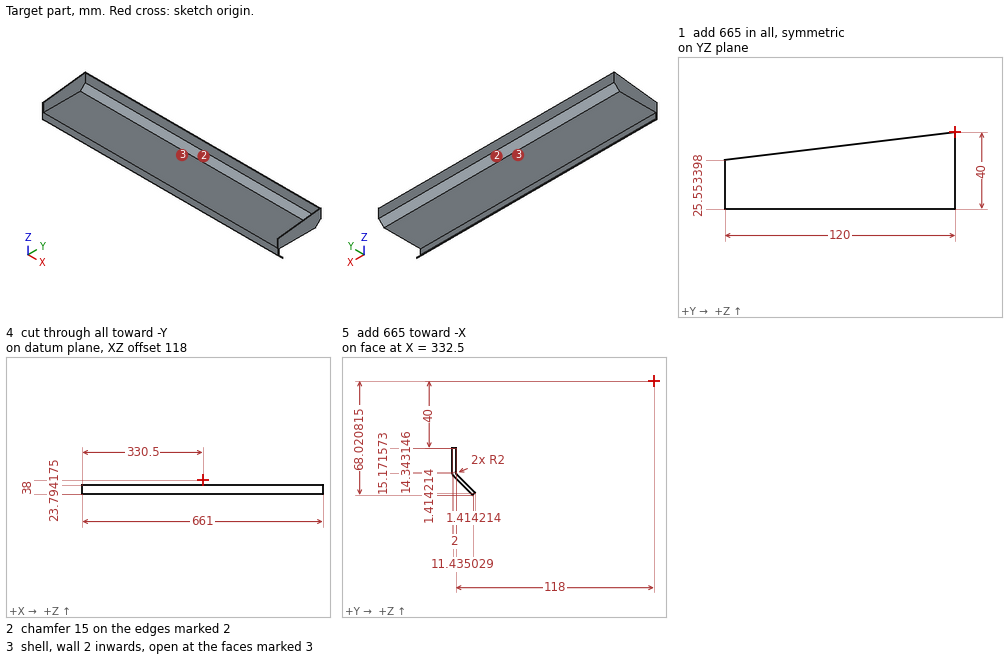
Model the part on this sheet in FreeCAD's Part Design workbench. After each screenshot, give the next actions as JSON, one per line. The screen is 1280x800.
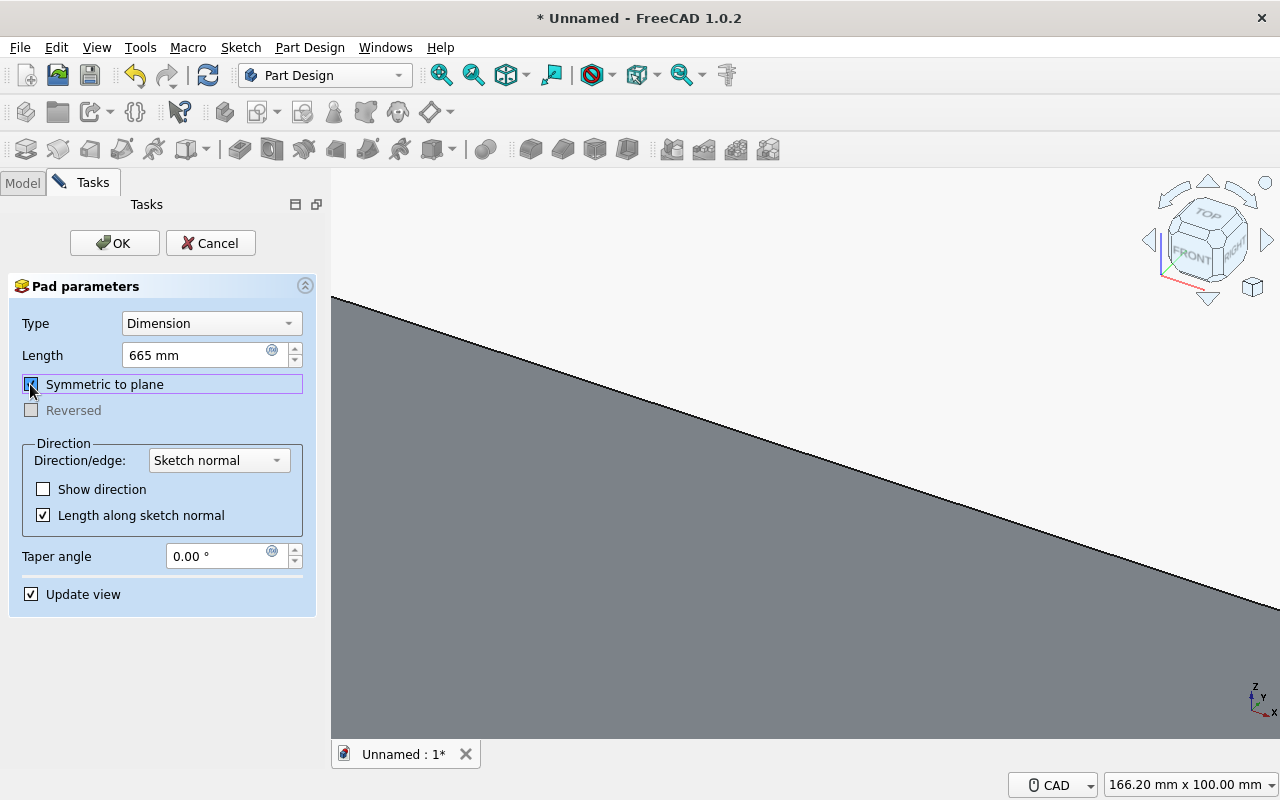
{"action": "left_click", "coordinate": [115, 243]}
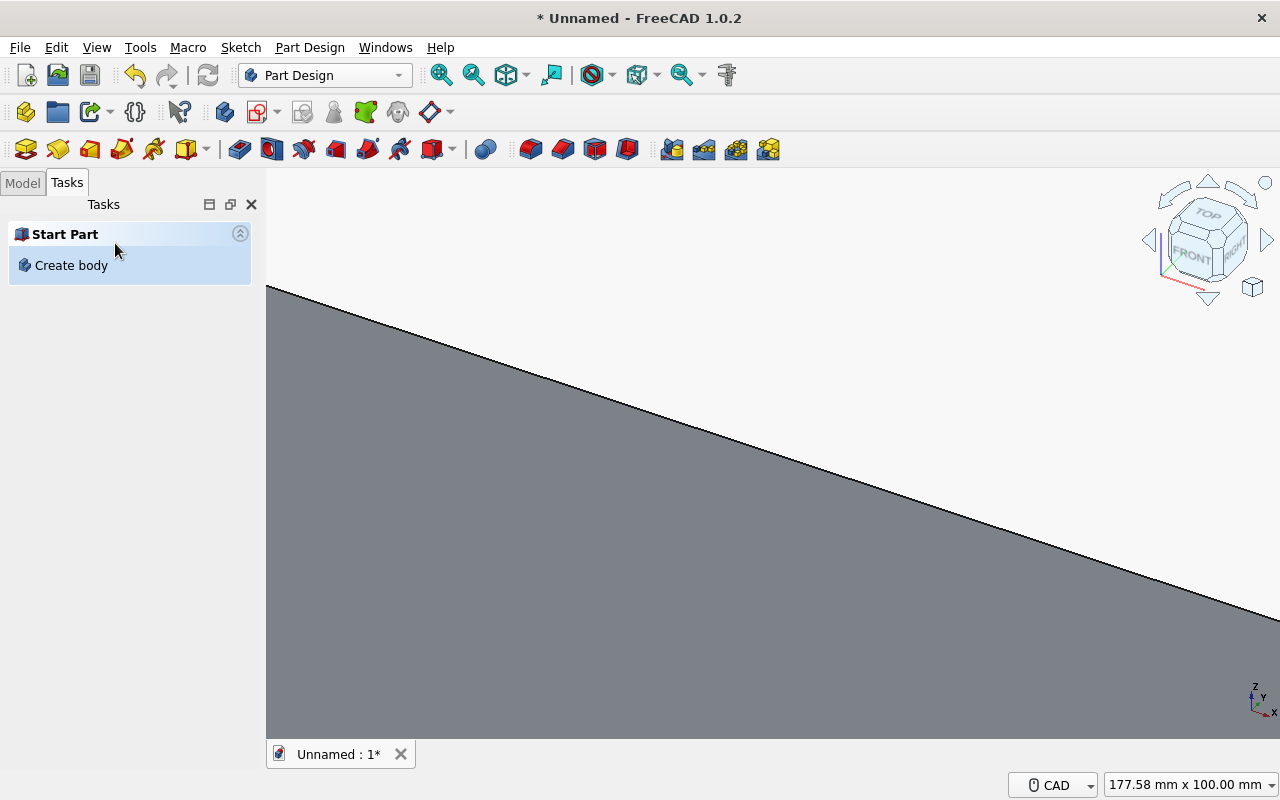
{"action": "left_click", "coordinate": [442, 76]}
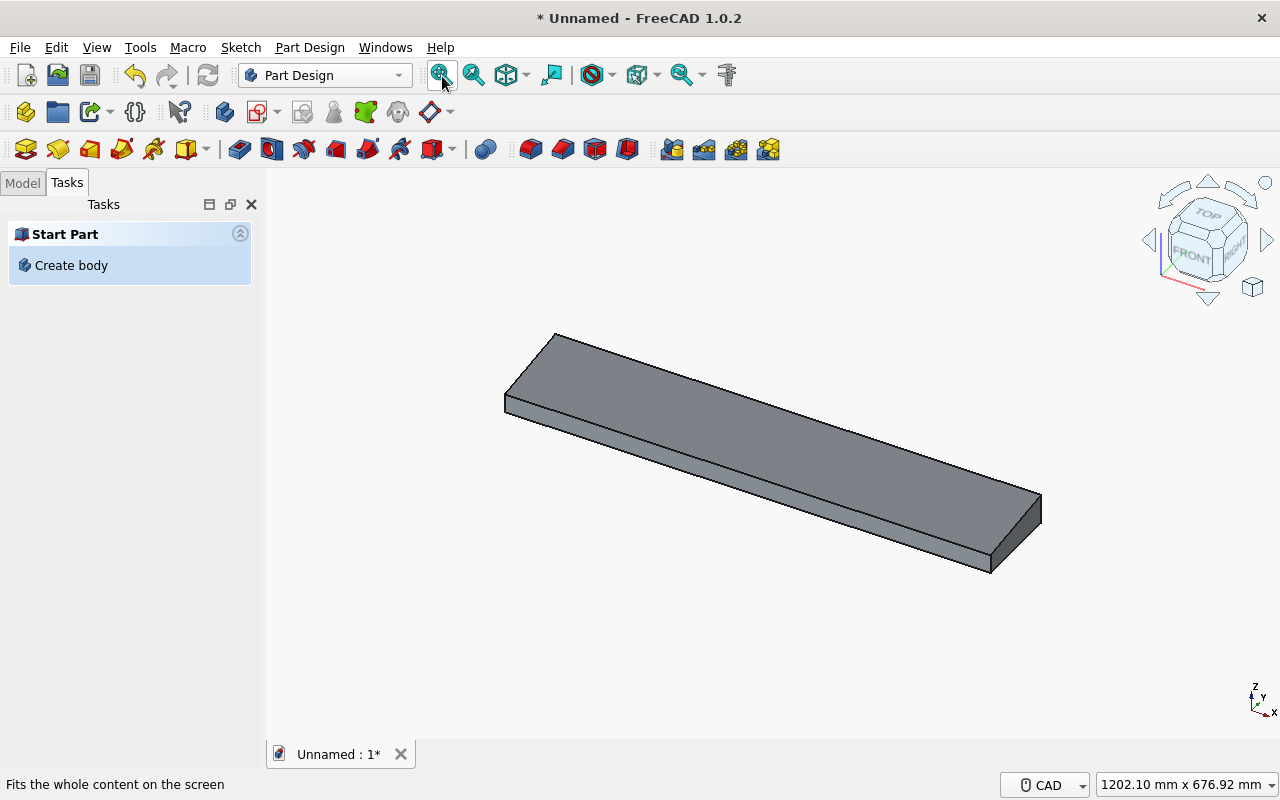
{"action": "key", "text": "0"}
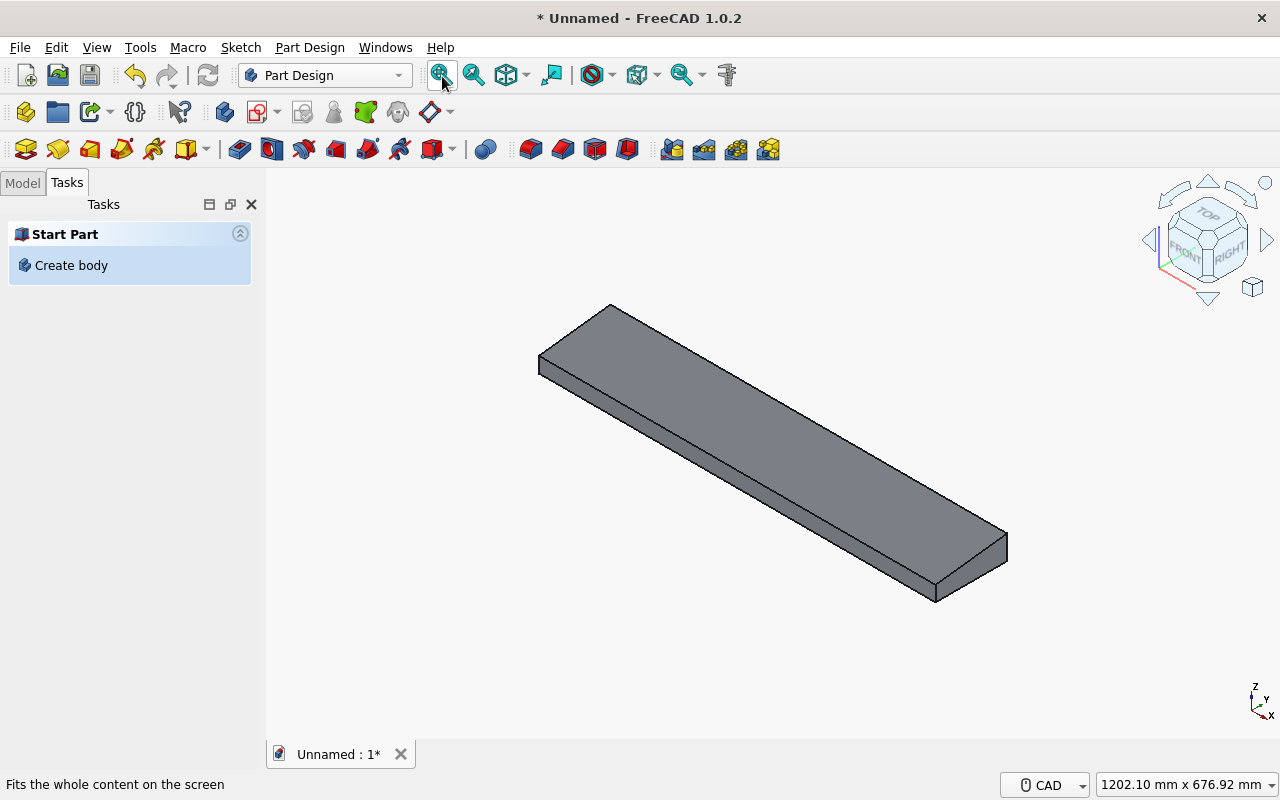
{"action": "key", "text": "2"}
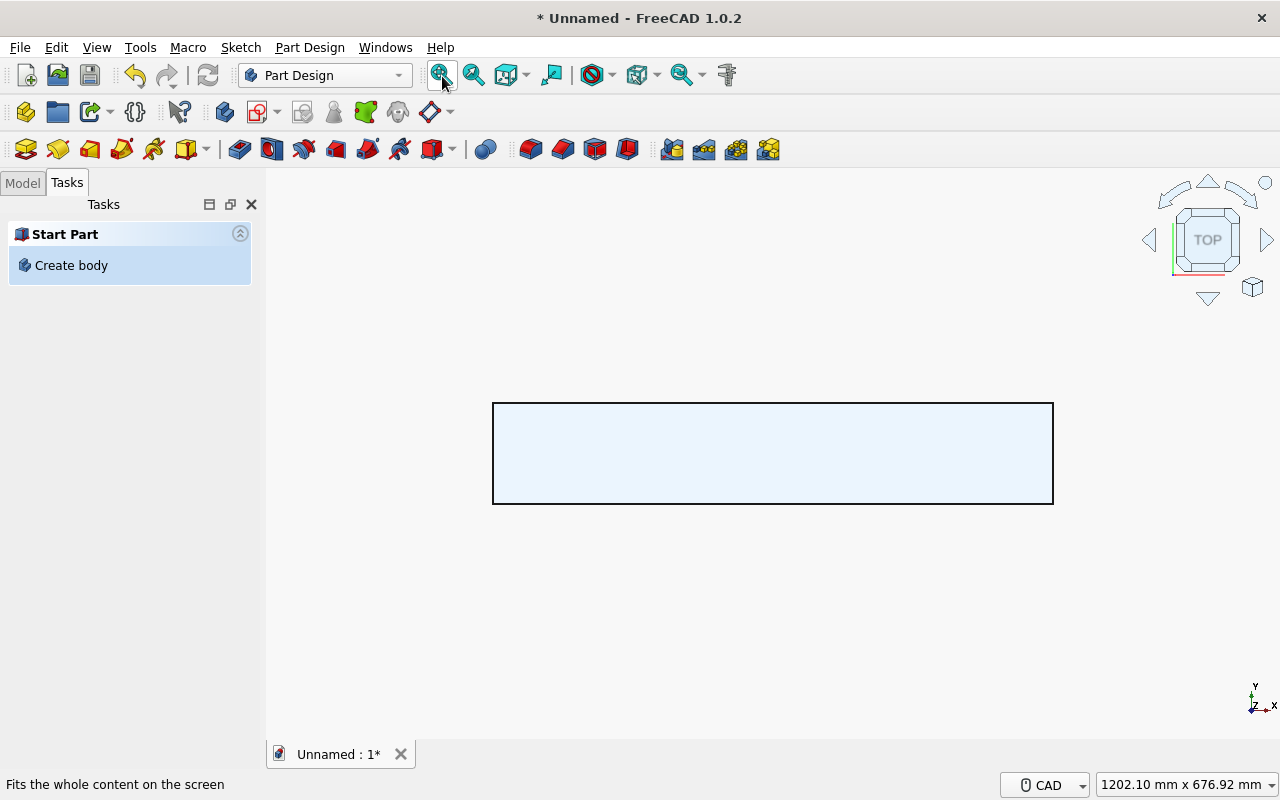
{"action": "key", "text": "1"}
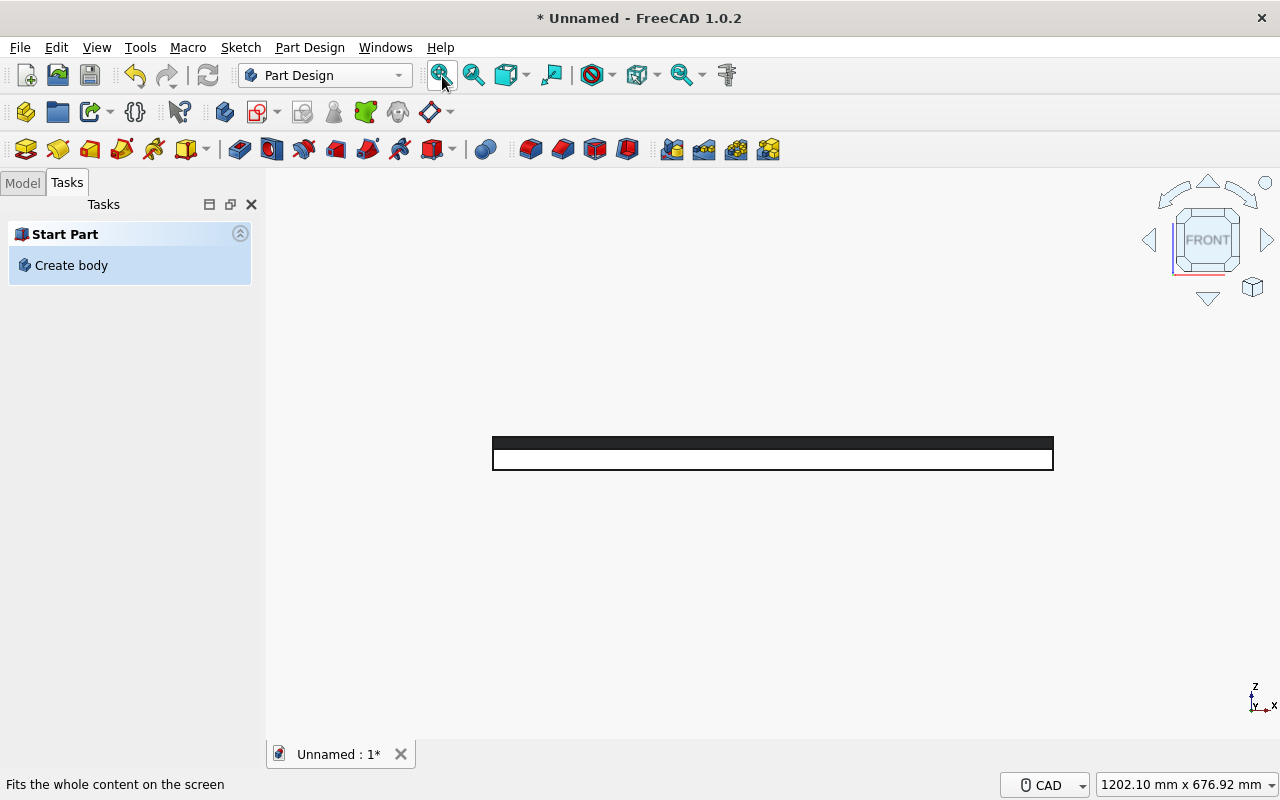
{"action": "key", "text": "3"}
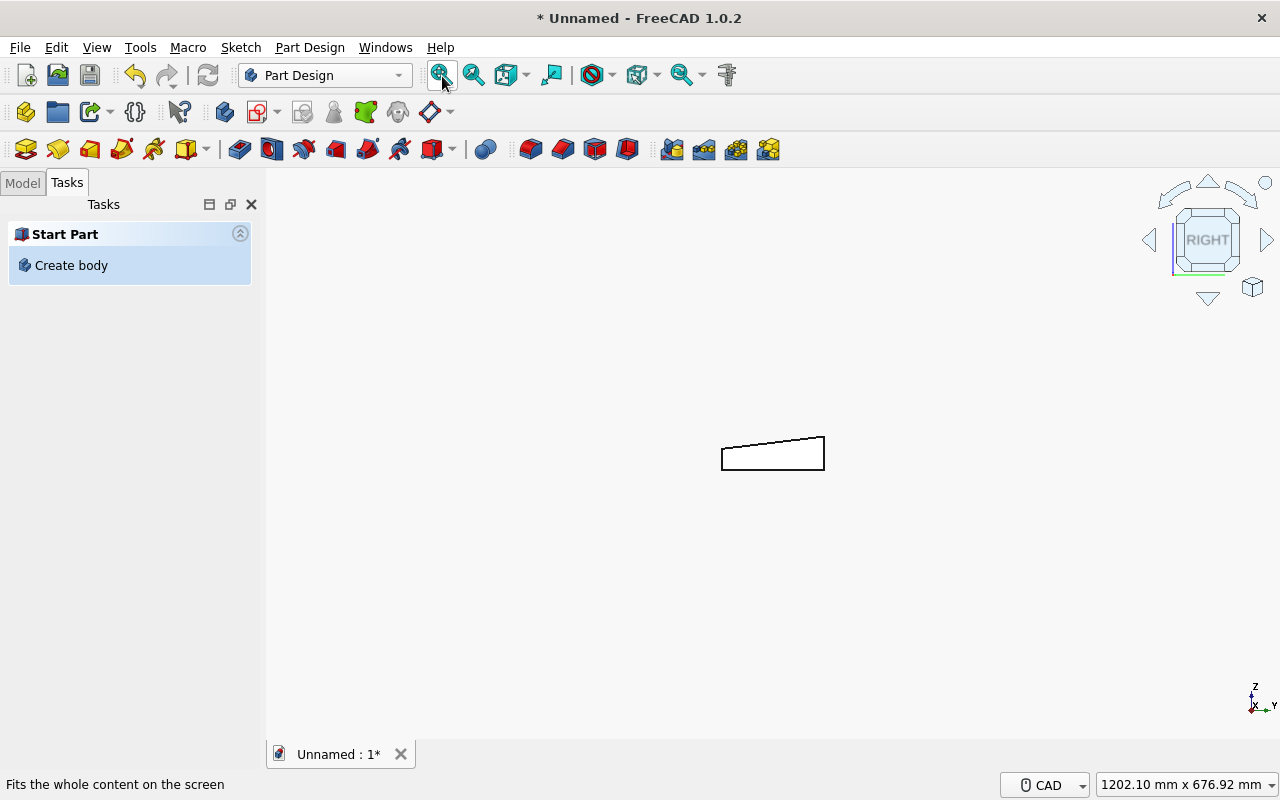
{"action": "key", "text": "v f"}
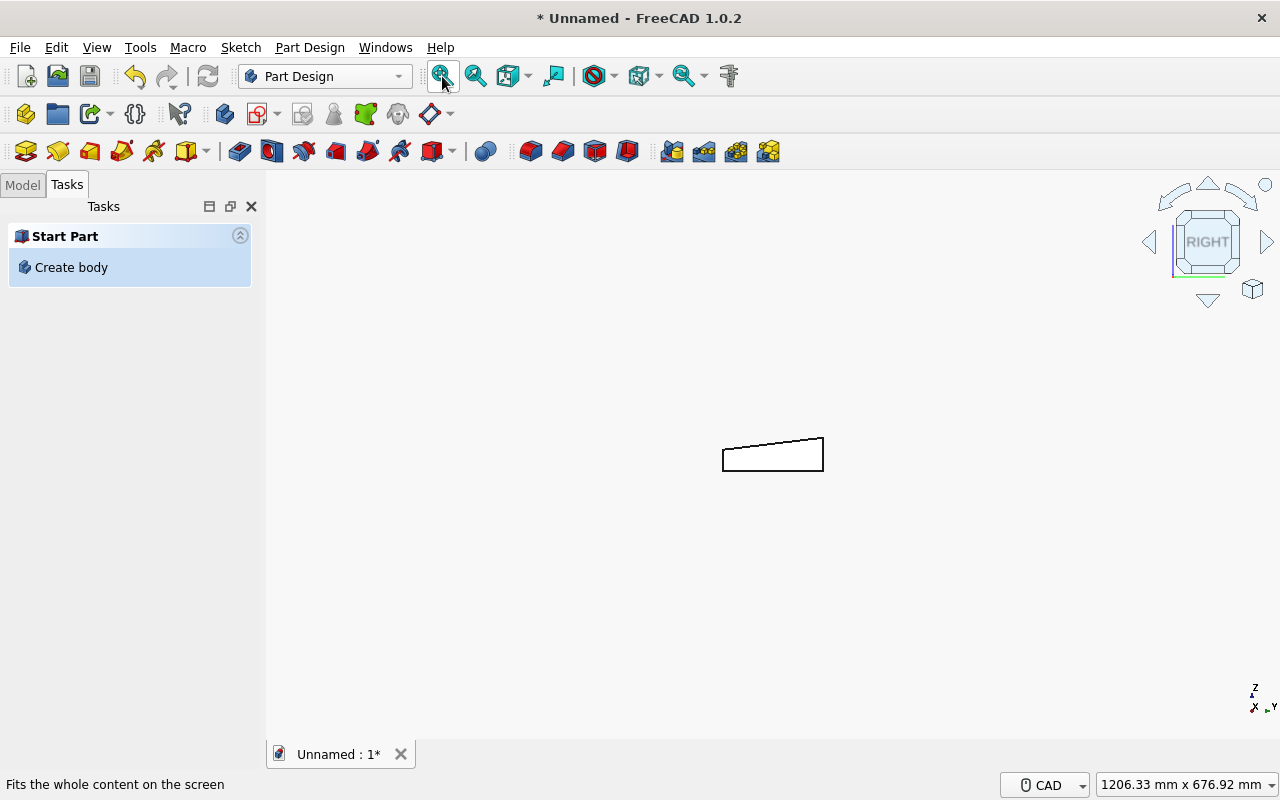
{"action": "key", "text": "5"}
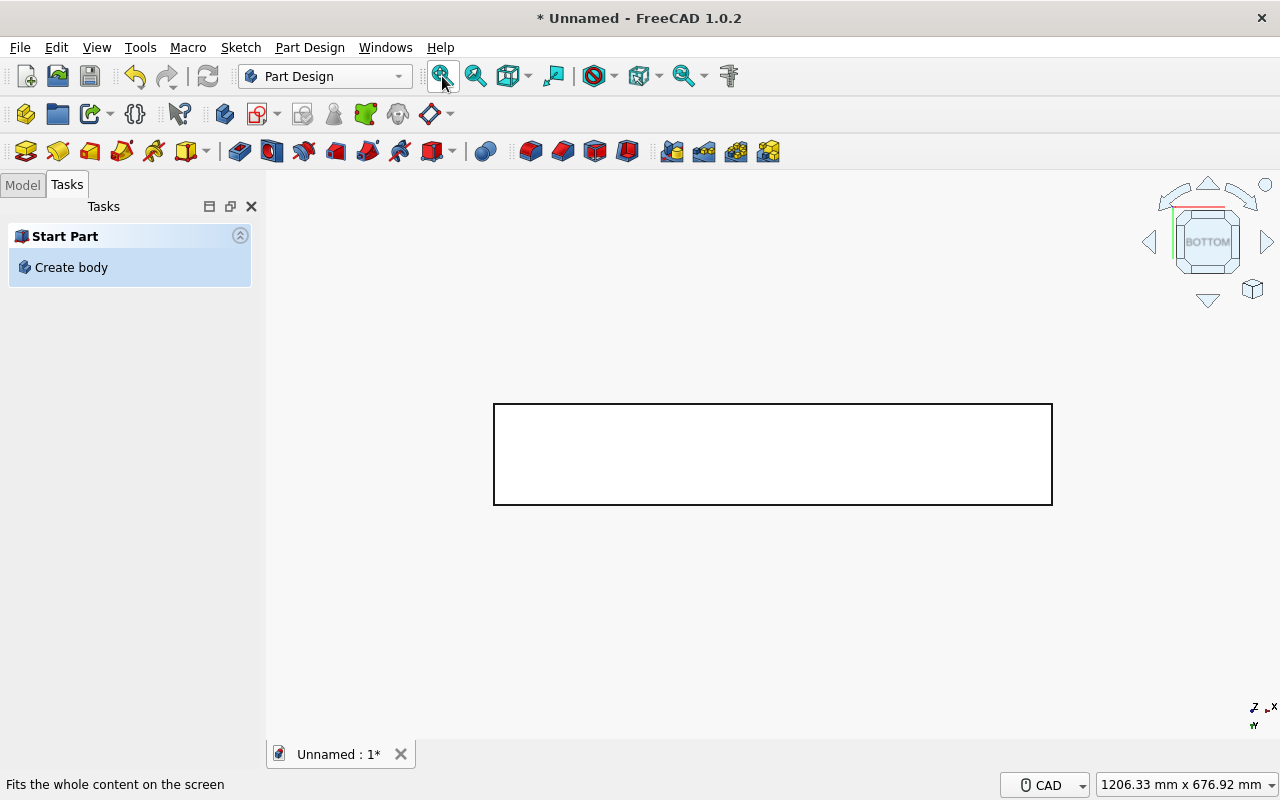
{"action": "left_click", "coordinate": [773, 504]}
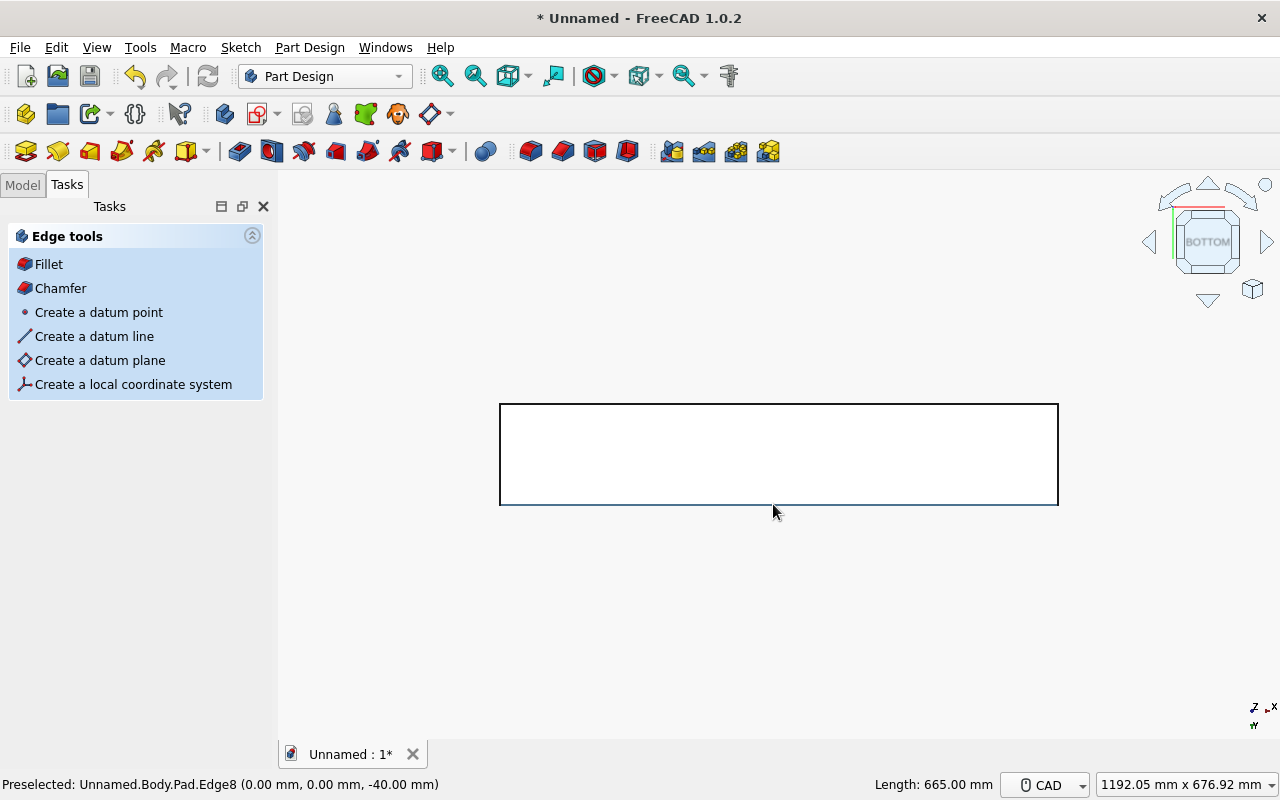
{"action": "left_click", "coordinate": [564, 152]}